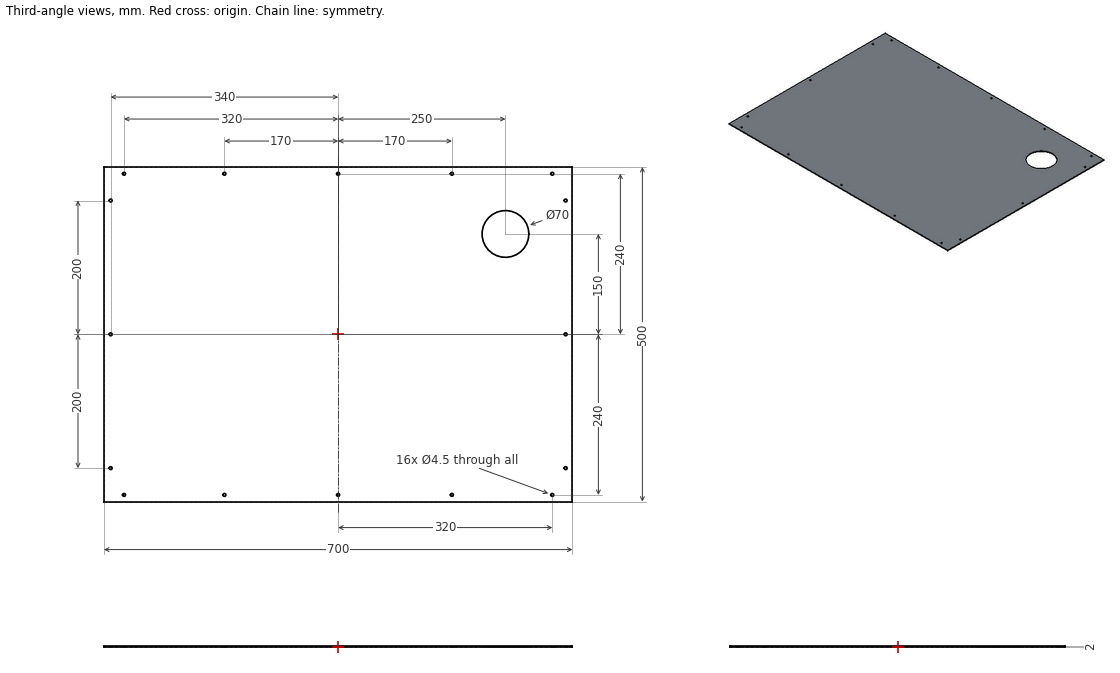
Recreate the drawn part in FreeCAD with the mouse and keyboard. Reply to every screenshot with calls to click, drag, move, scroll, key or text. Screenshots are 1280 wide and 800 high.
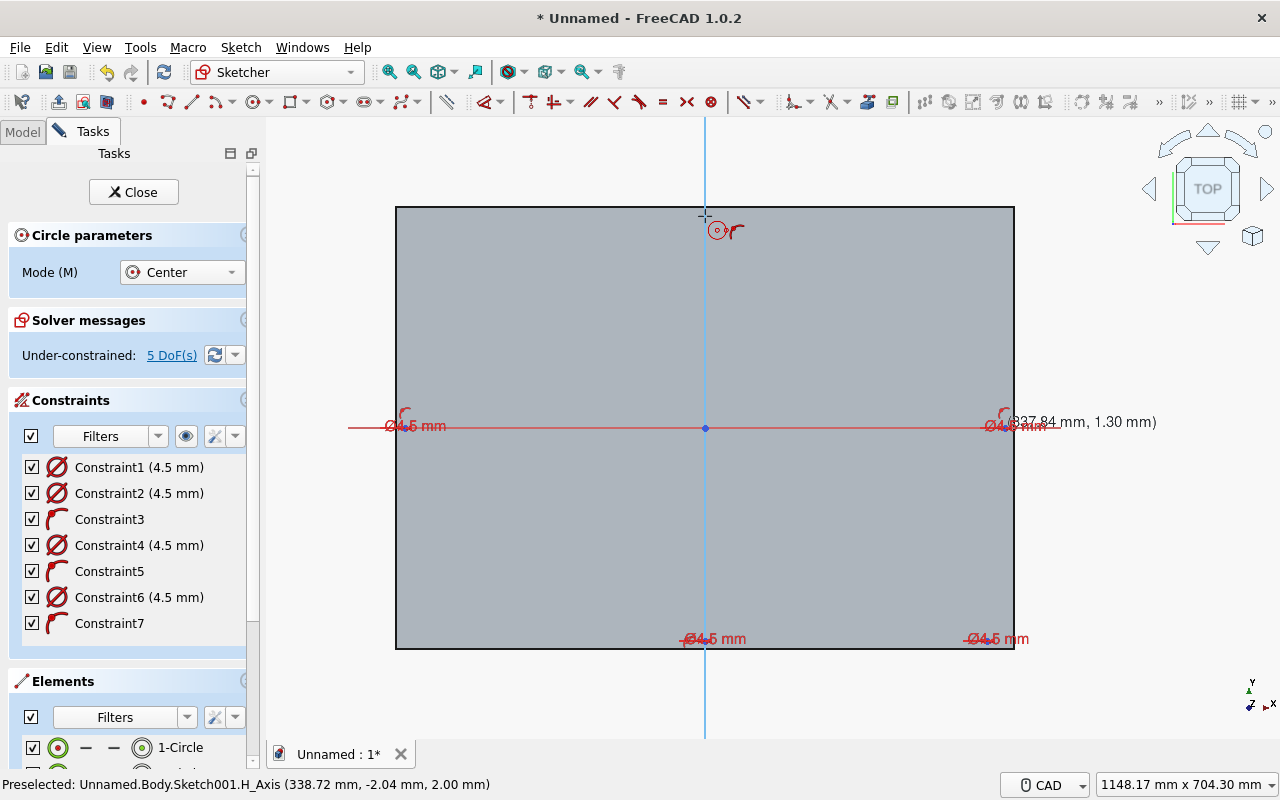
click(705, 216)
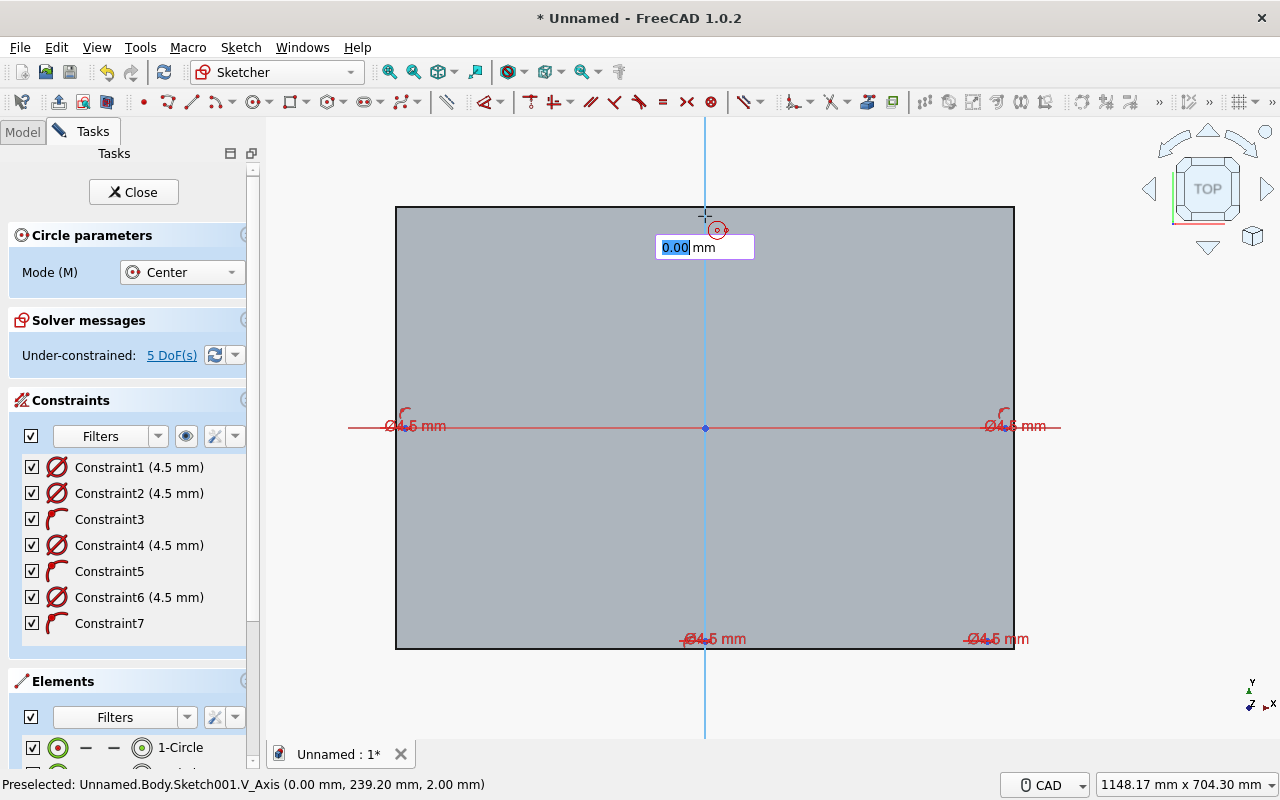
scroll(707, 216, up, 11)
move(702, 211)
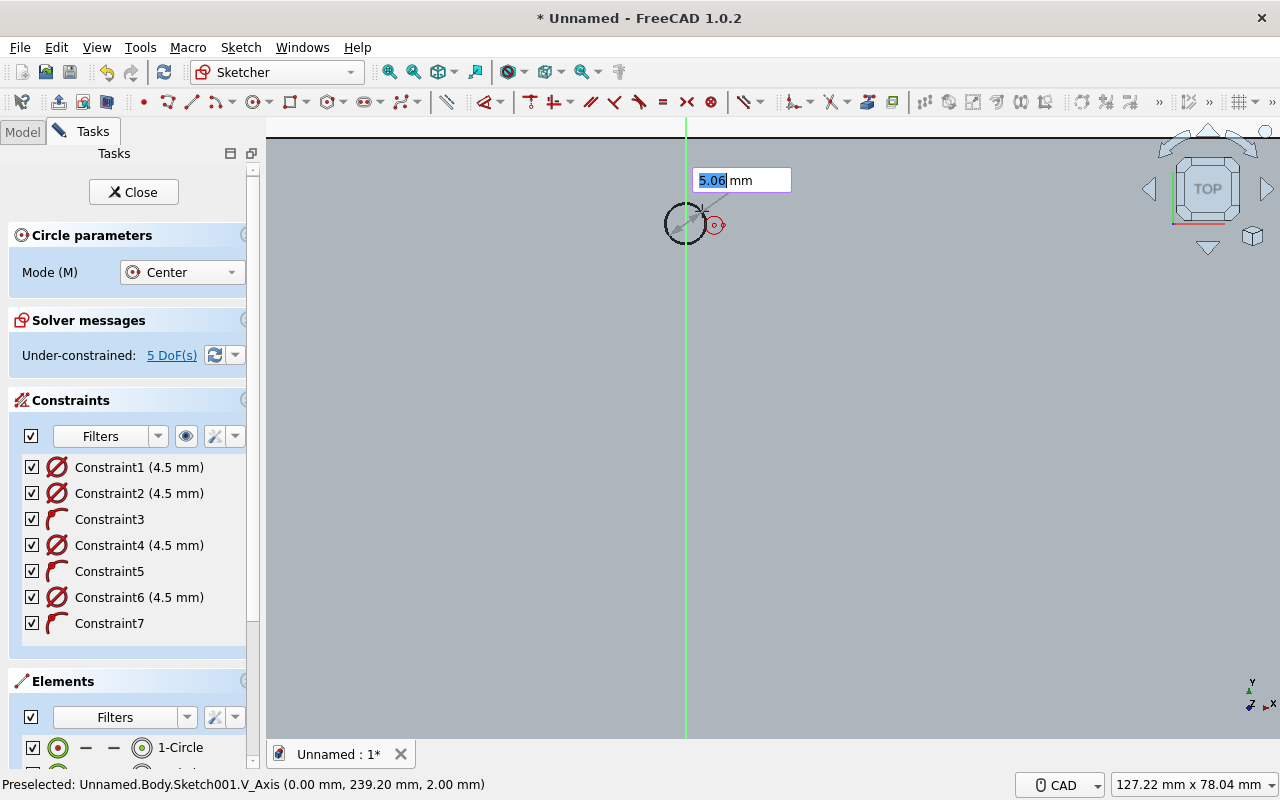
text(4.5)
key(Return)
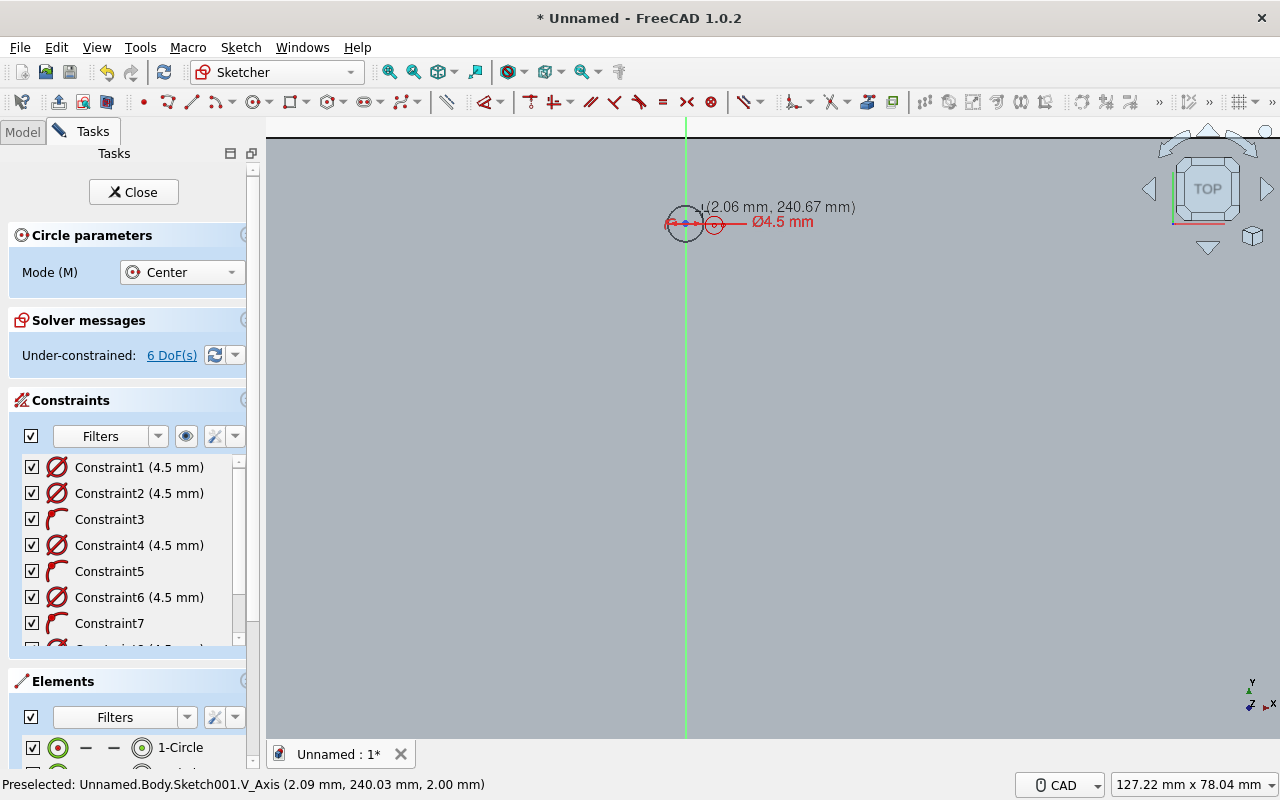
scroll(707, 216, down, 11)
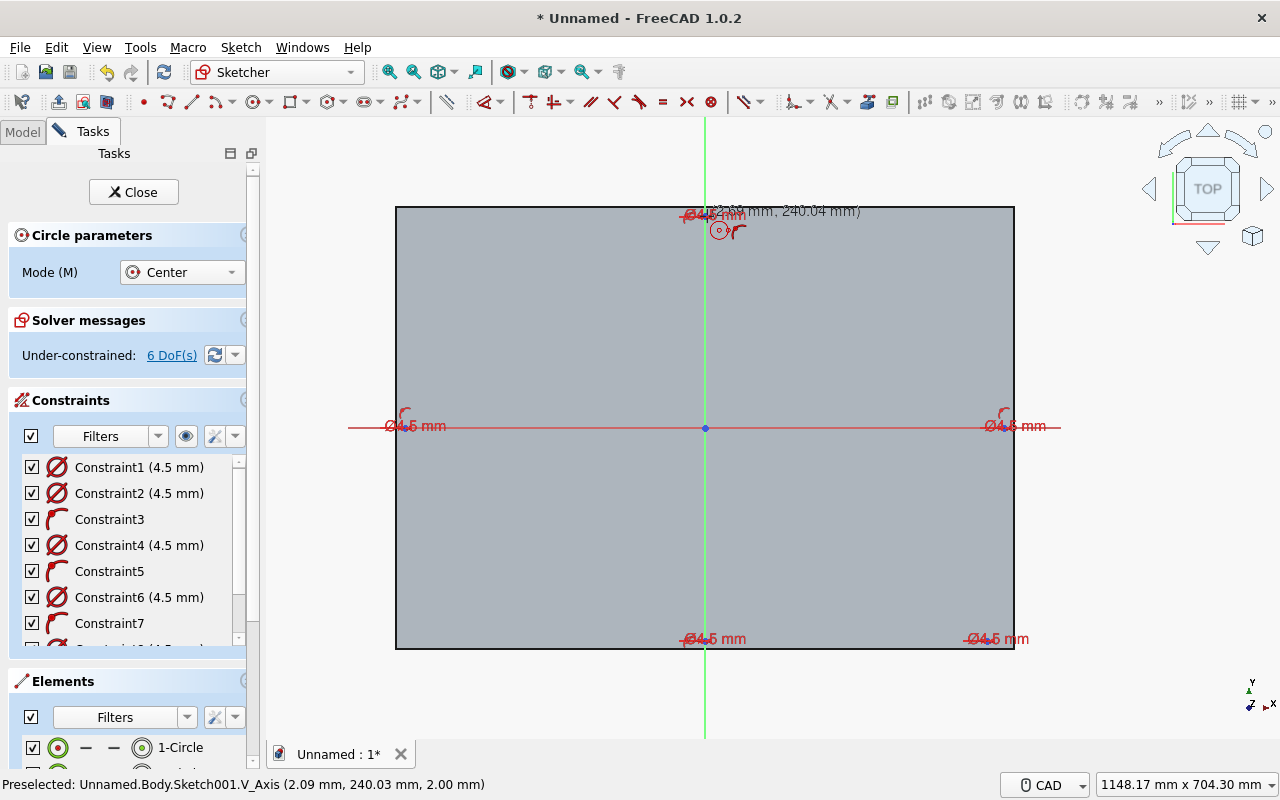
scroll(555, 216, up, 13)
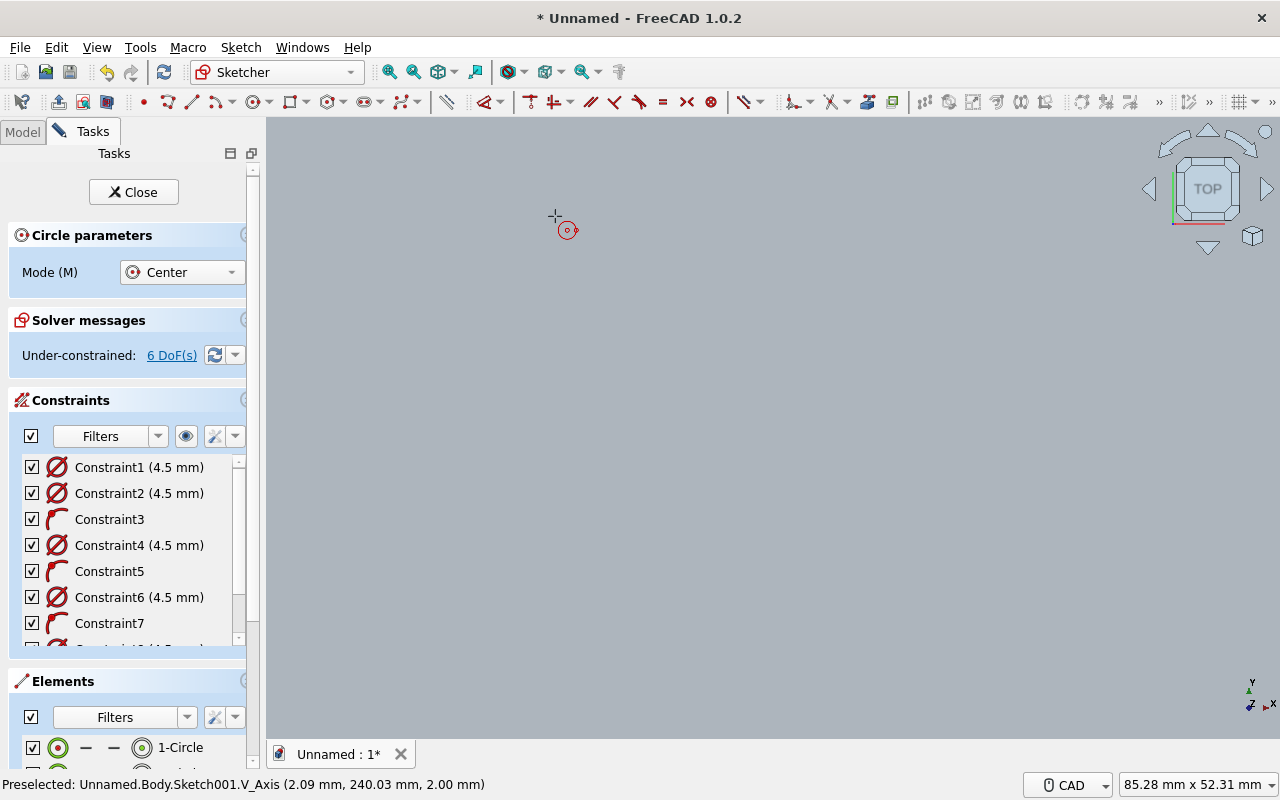
scroll(555, 216, down, 13)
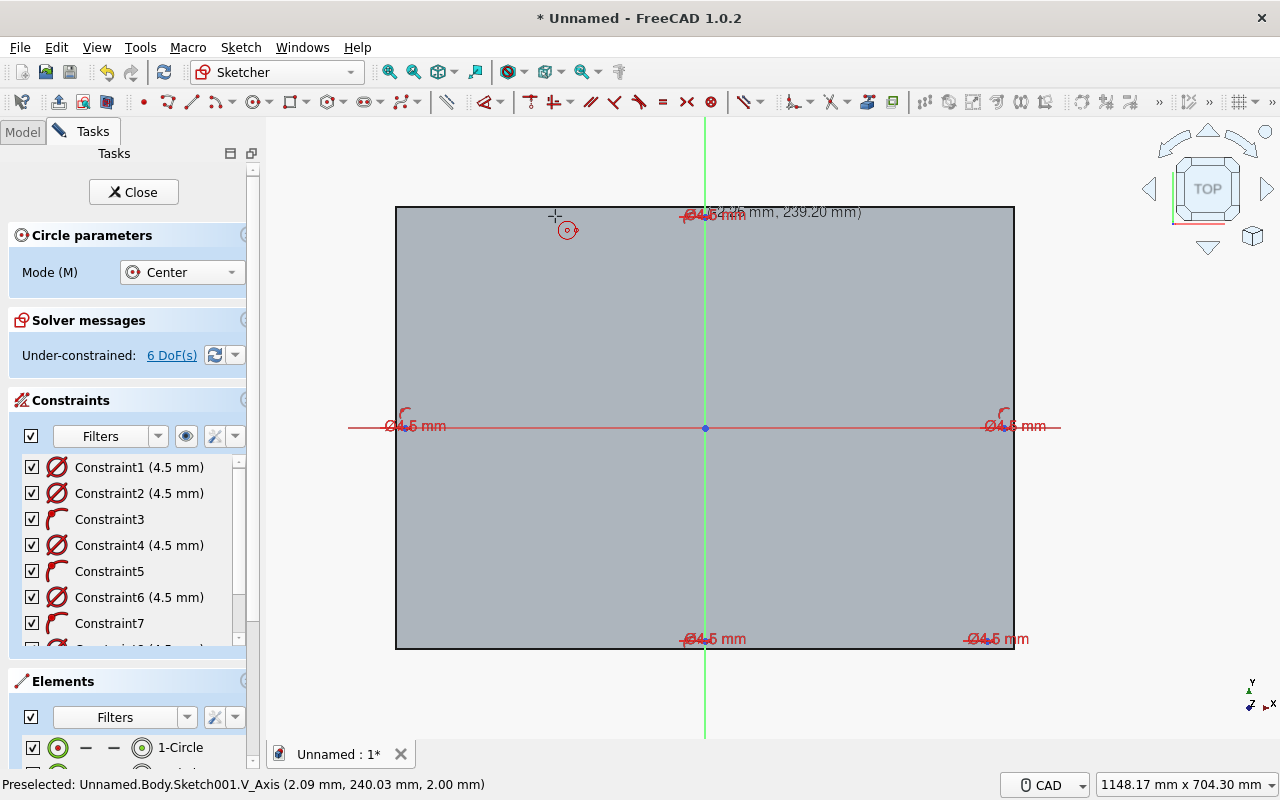
click(555, 216)
move(556, 215)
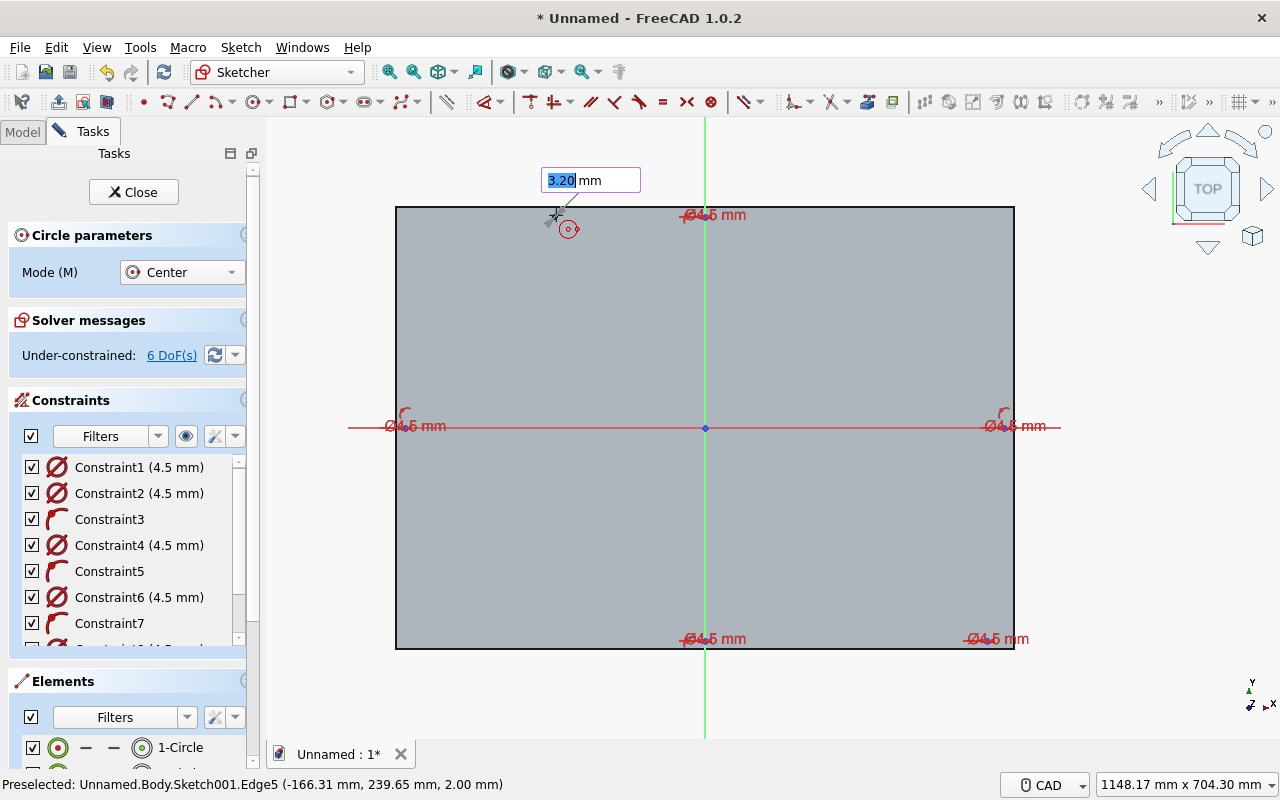
text(4.5)
key(Return)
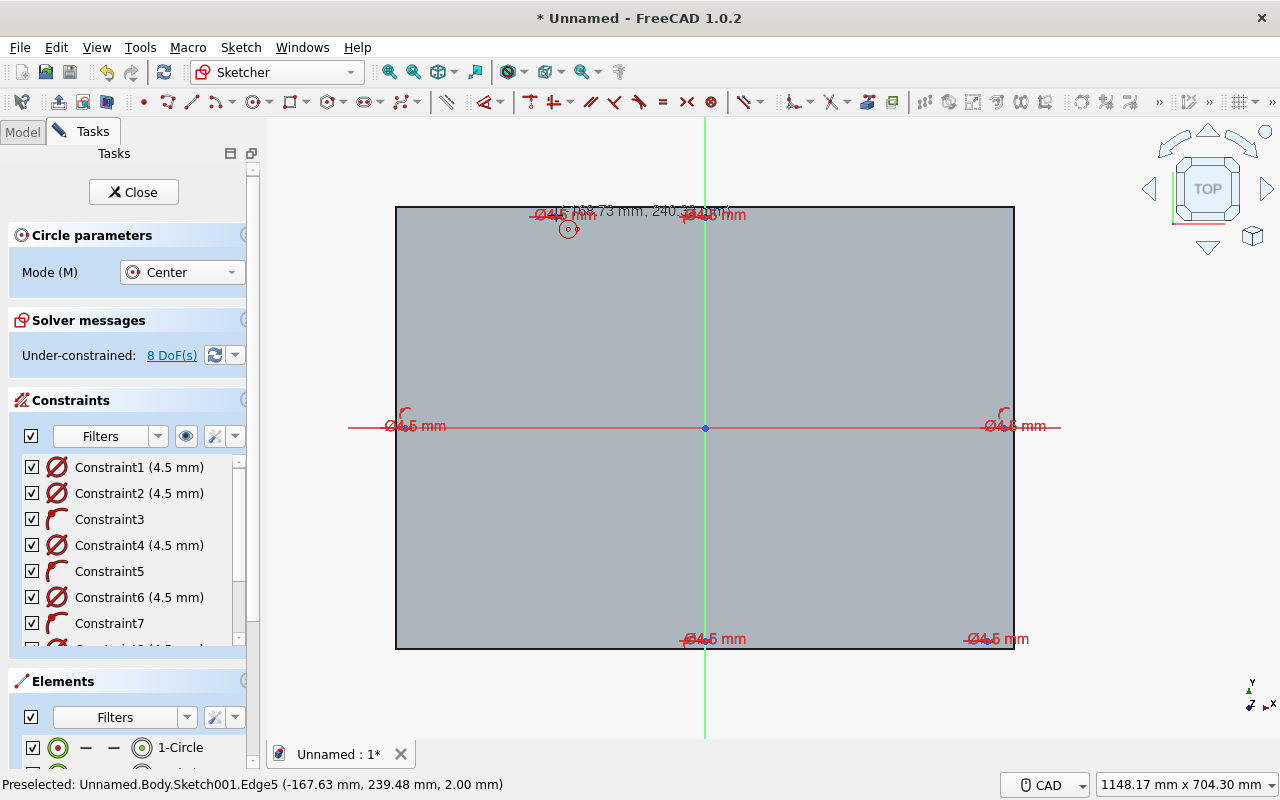
scroll(855, 216, up, 13)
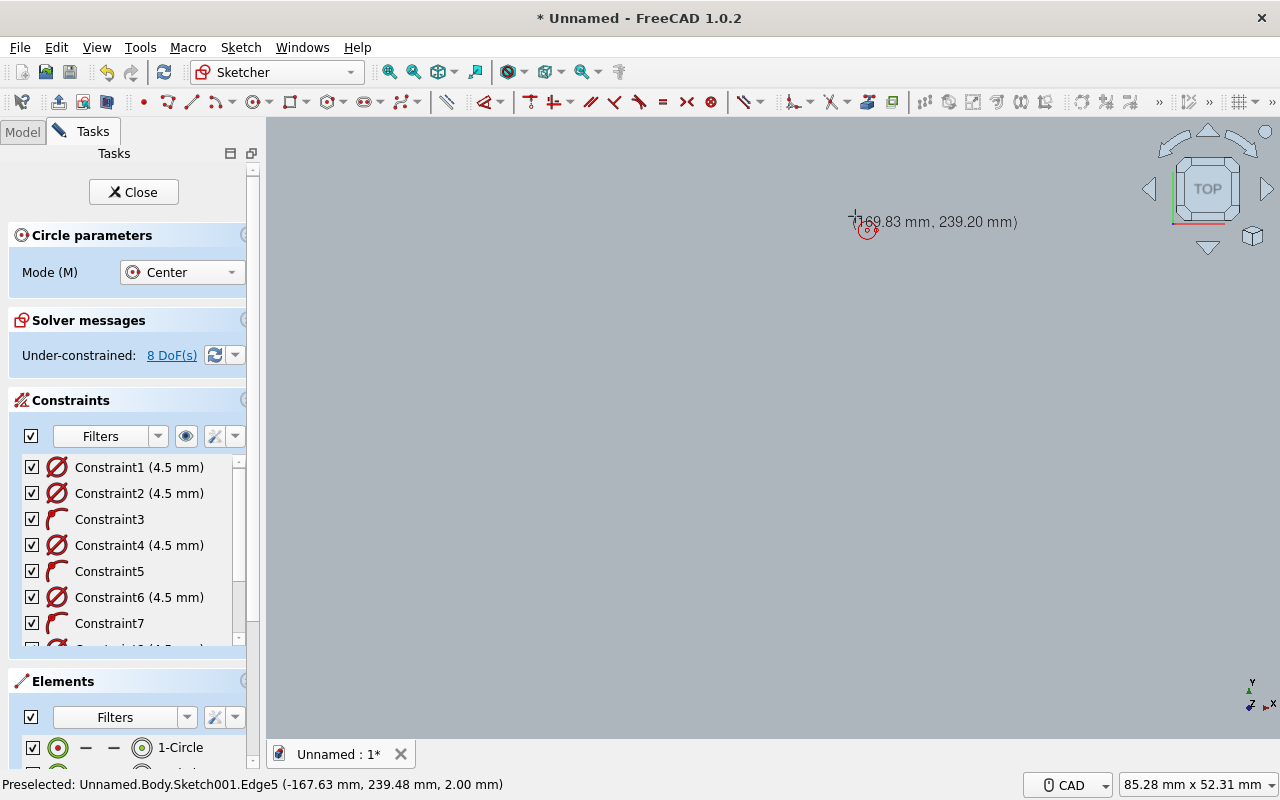
scroll(855, 216, down, 13)